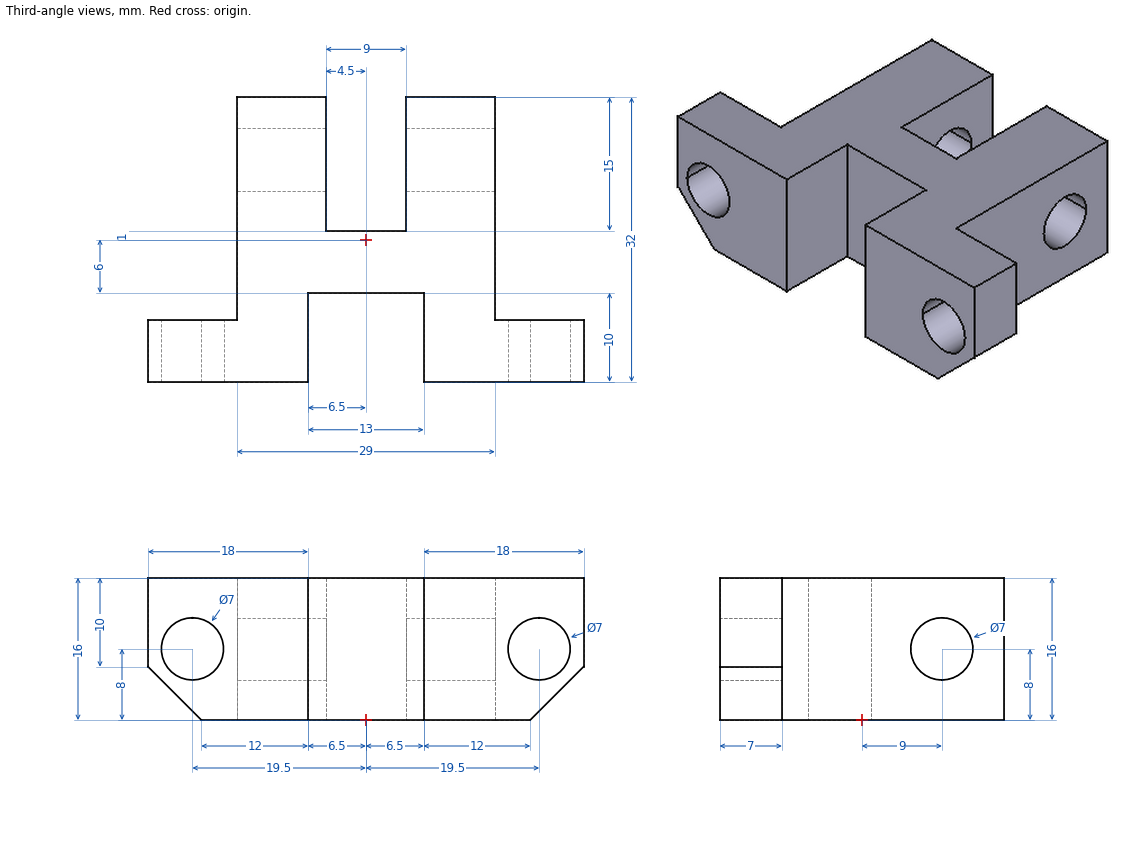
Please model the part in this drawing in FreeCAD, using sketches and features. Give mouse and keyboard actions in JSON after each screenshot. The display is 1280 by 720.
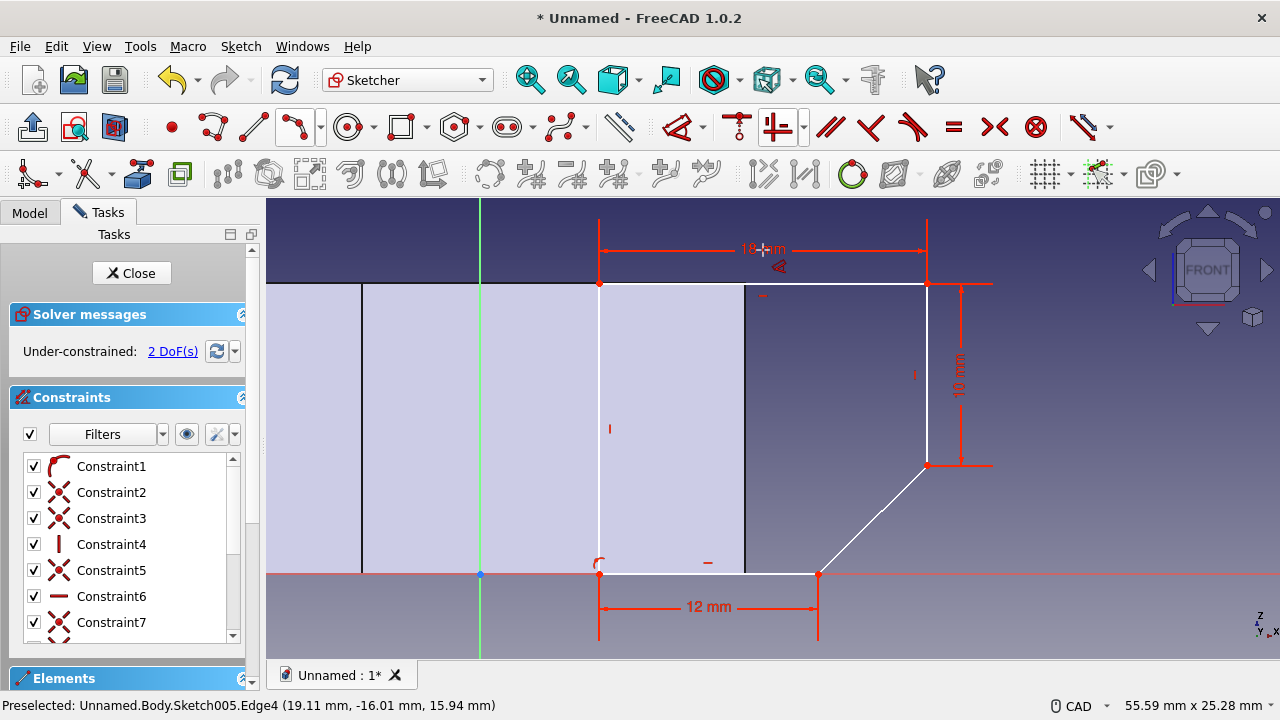
{"action": "left_click", "coordinate": [599, 371]}
{"action": "left_click", "coordinate": [565, 429]}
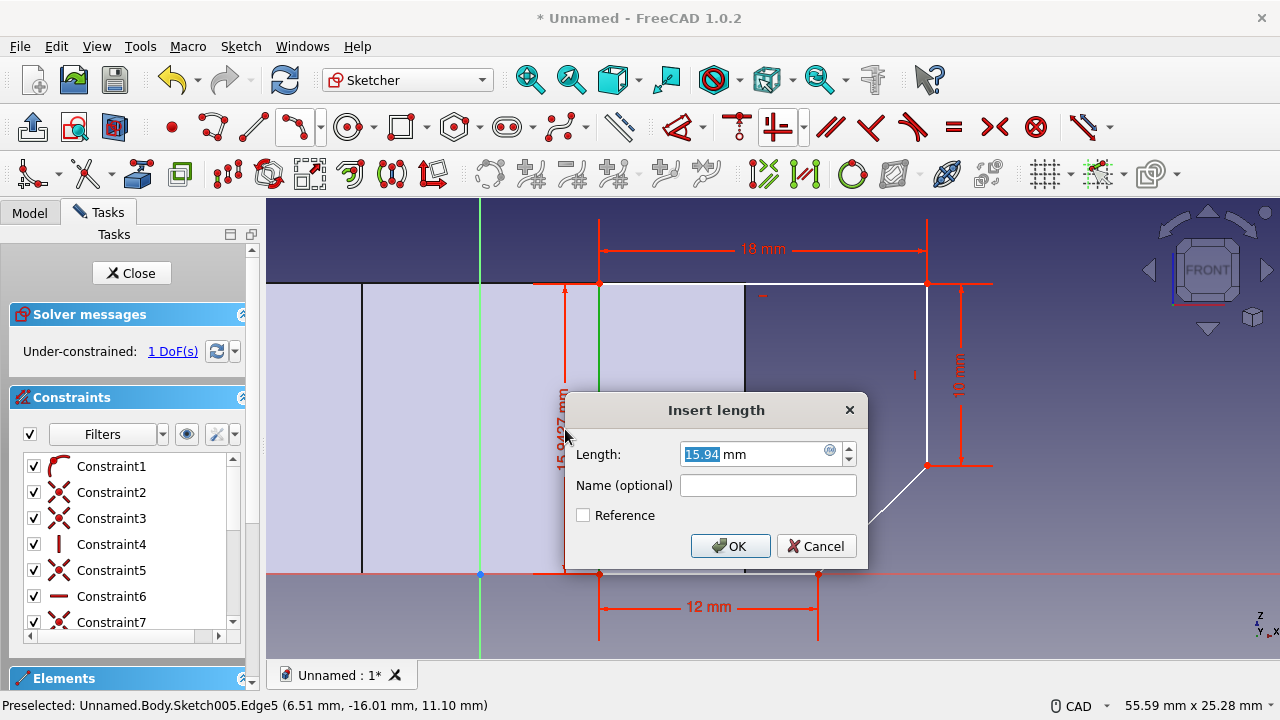
{"action": "type", "text": "16"}
{"action": "key", "text": "Return"}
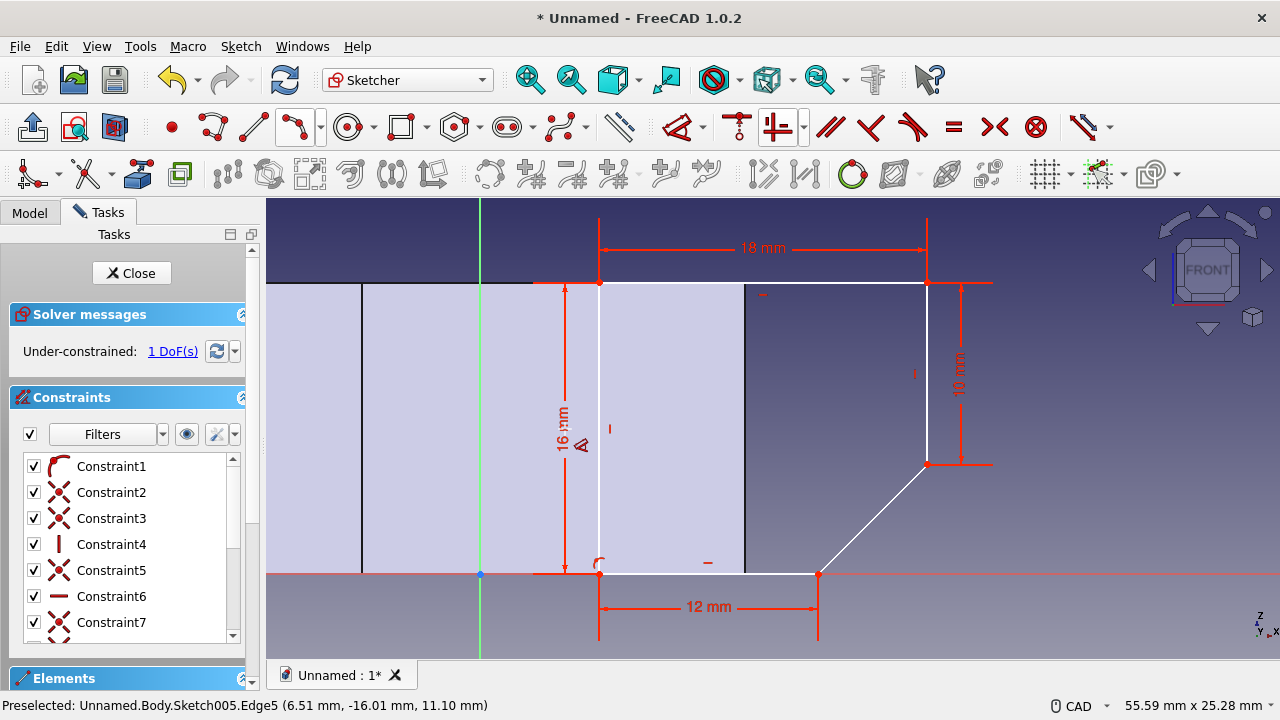
{"action": "left_click", "coordinate": [599, 574]}
{"action": "left_click", "coordinate": [540, 608]}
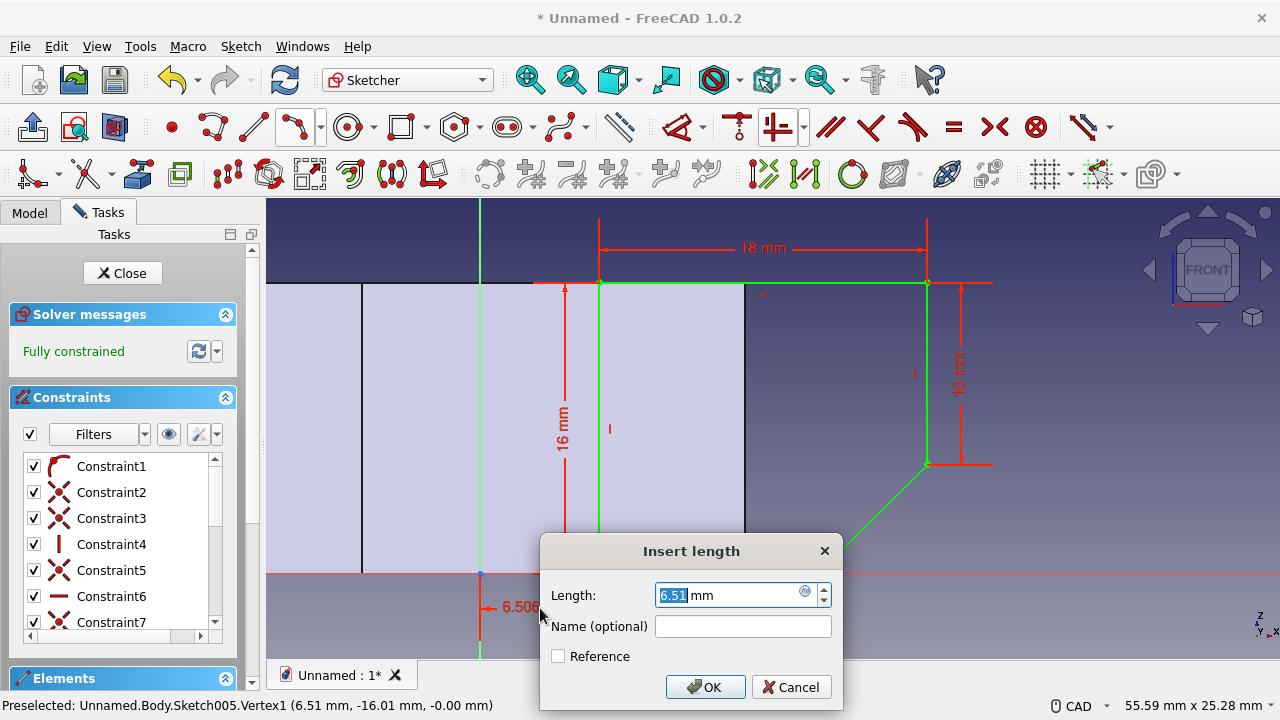
{"action": "type", "text": "6.5"}
{"action": "key", "text": "Return"}
{"action": "key", "text": "Escape"}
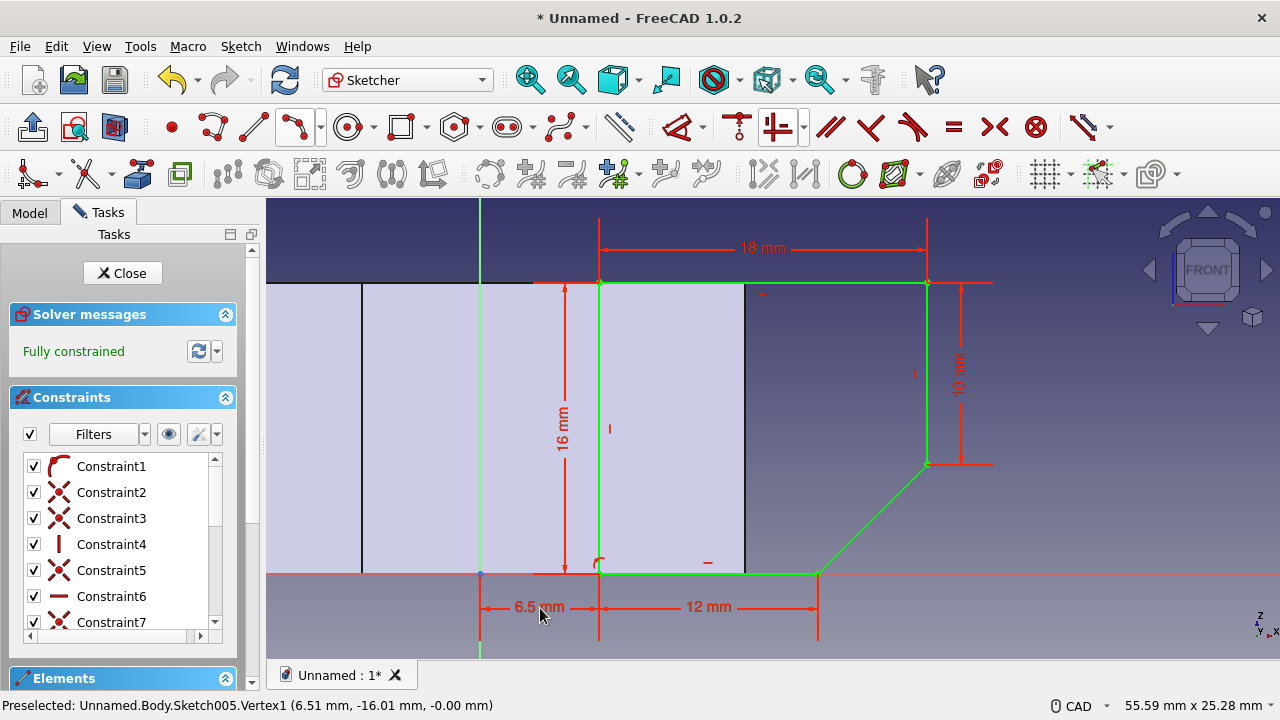
{"action": "left_click", "coordinate": [123, 273]}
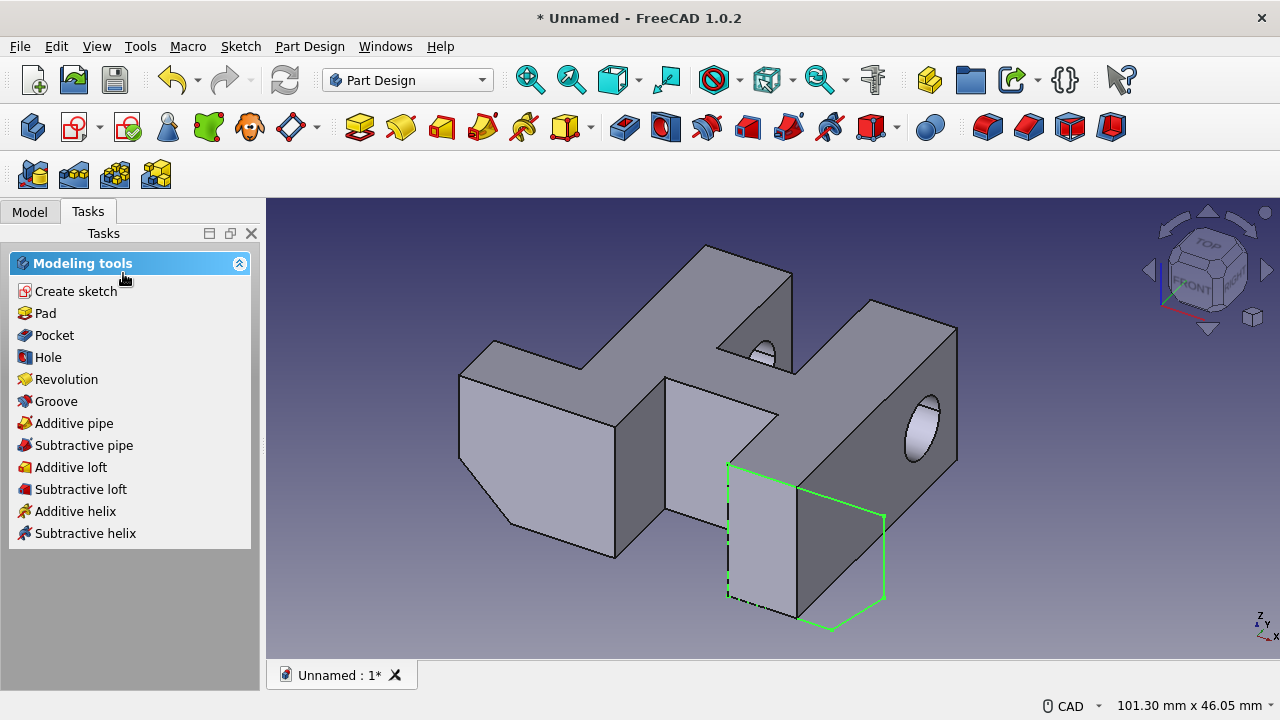
{"action": "left_click", "coordinate": [360, 128]}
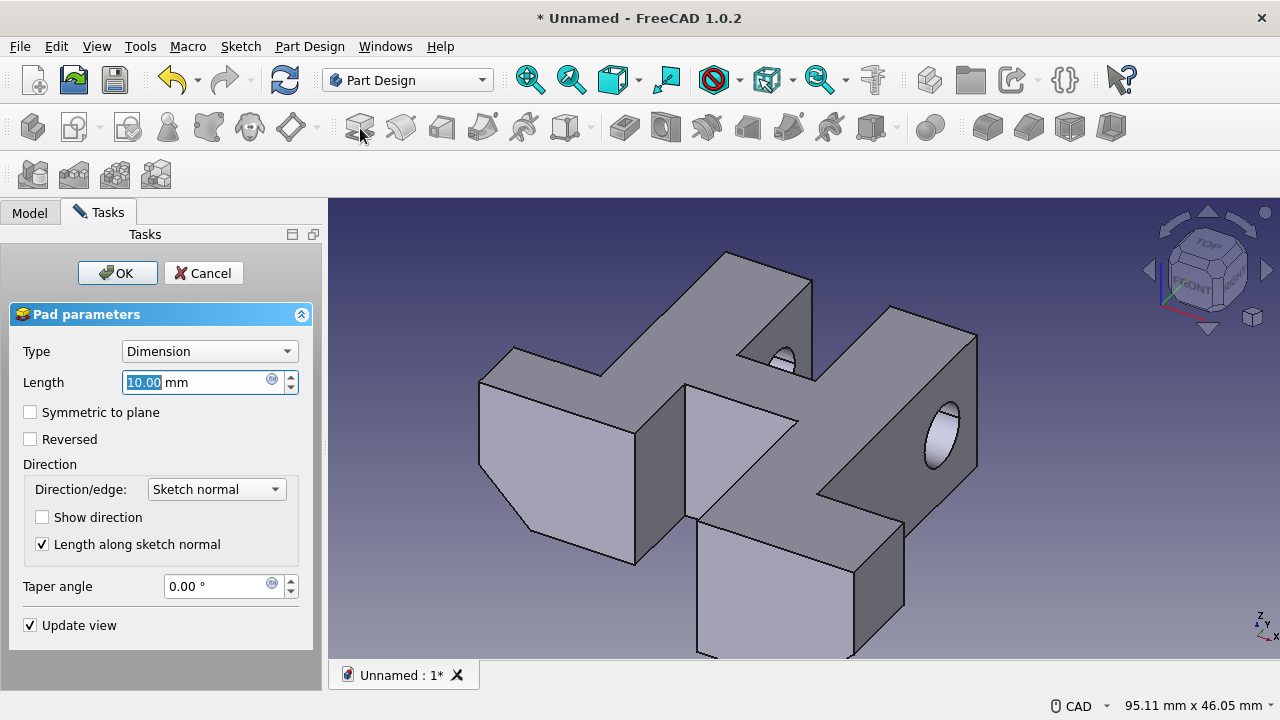
{"action": "type", "text": "7"}
{"action": "key", "text": "Tab"}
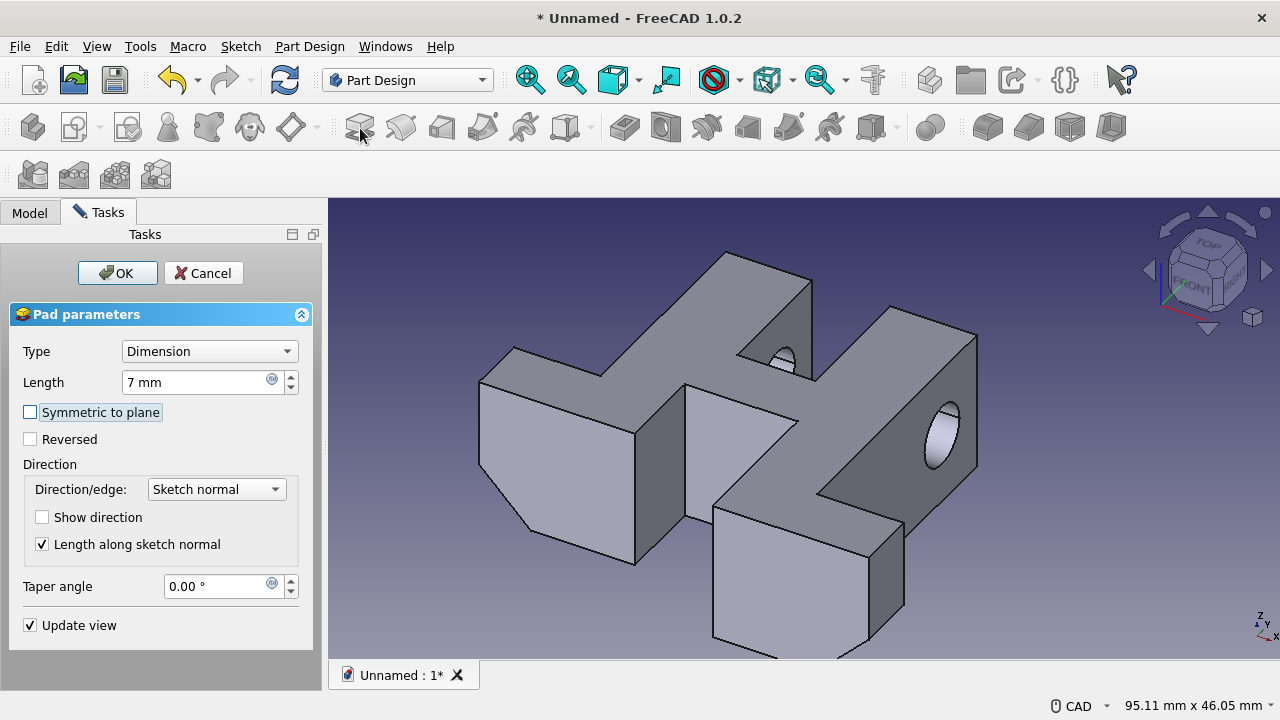
{"action": "left_click", "coordinate": [31, 439]}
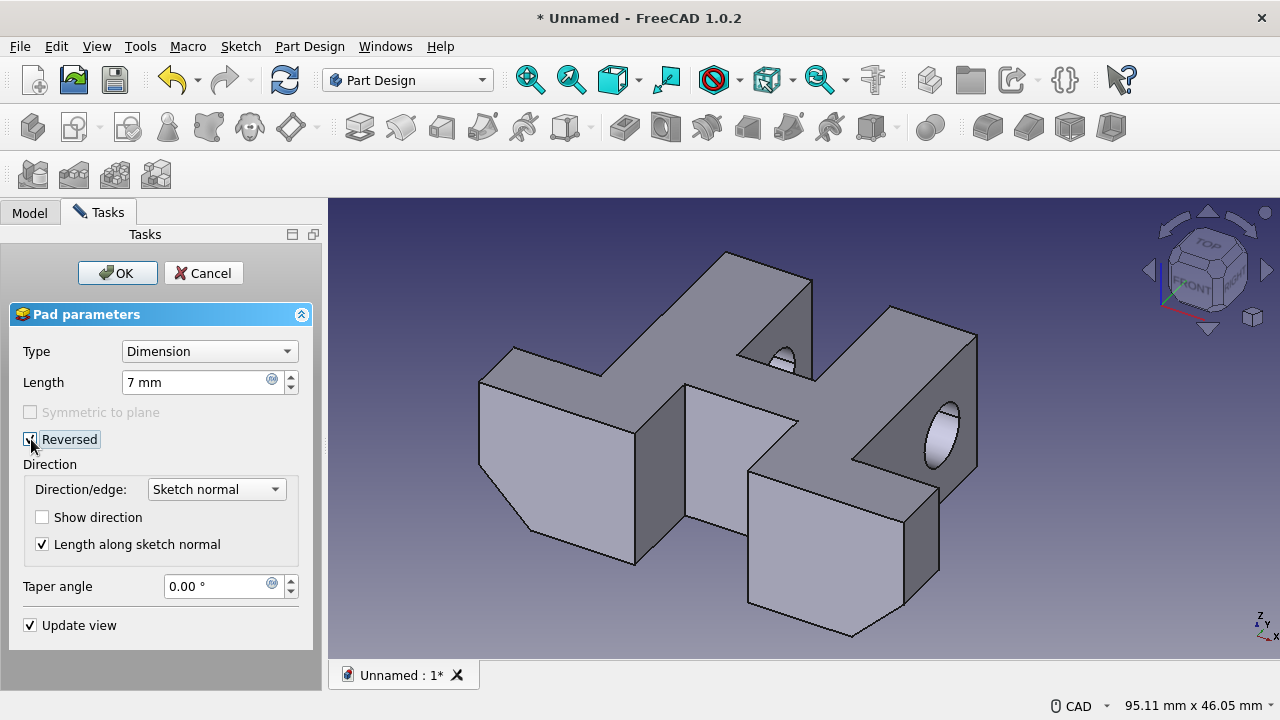
{"action": "left_click", "coordinate": [118, 273]}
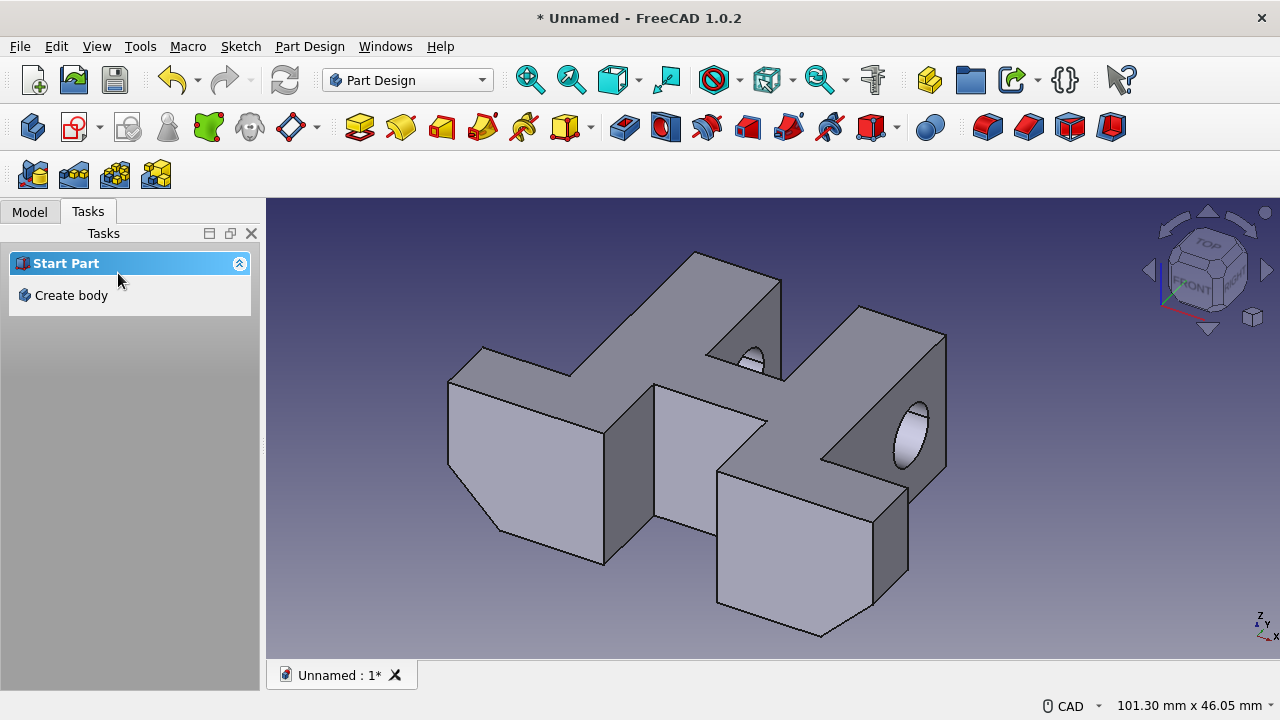
{"action": "key", "text": "4"}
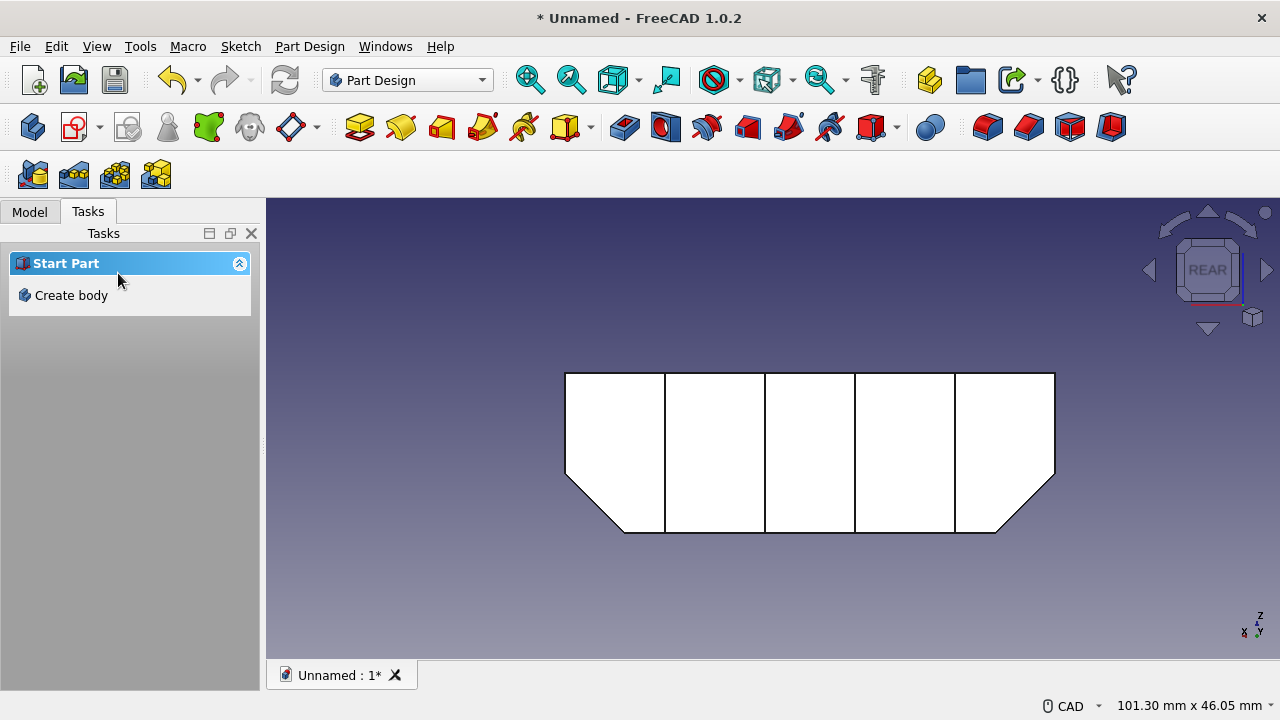
{"action": "left_click", "coordinate": [1005, 429]}